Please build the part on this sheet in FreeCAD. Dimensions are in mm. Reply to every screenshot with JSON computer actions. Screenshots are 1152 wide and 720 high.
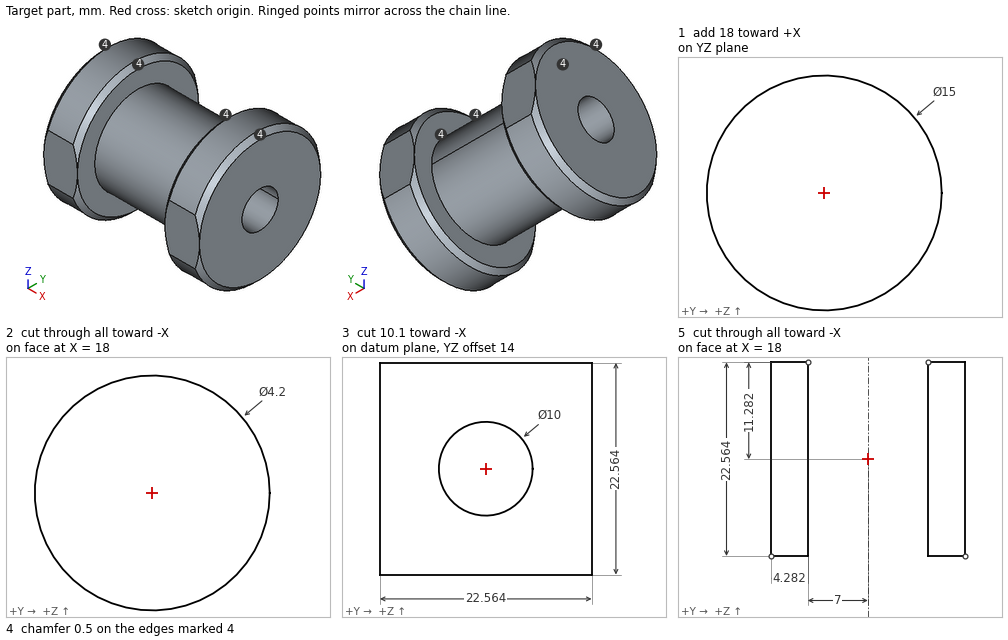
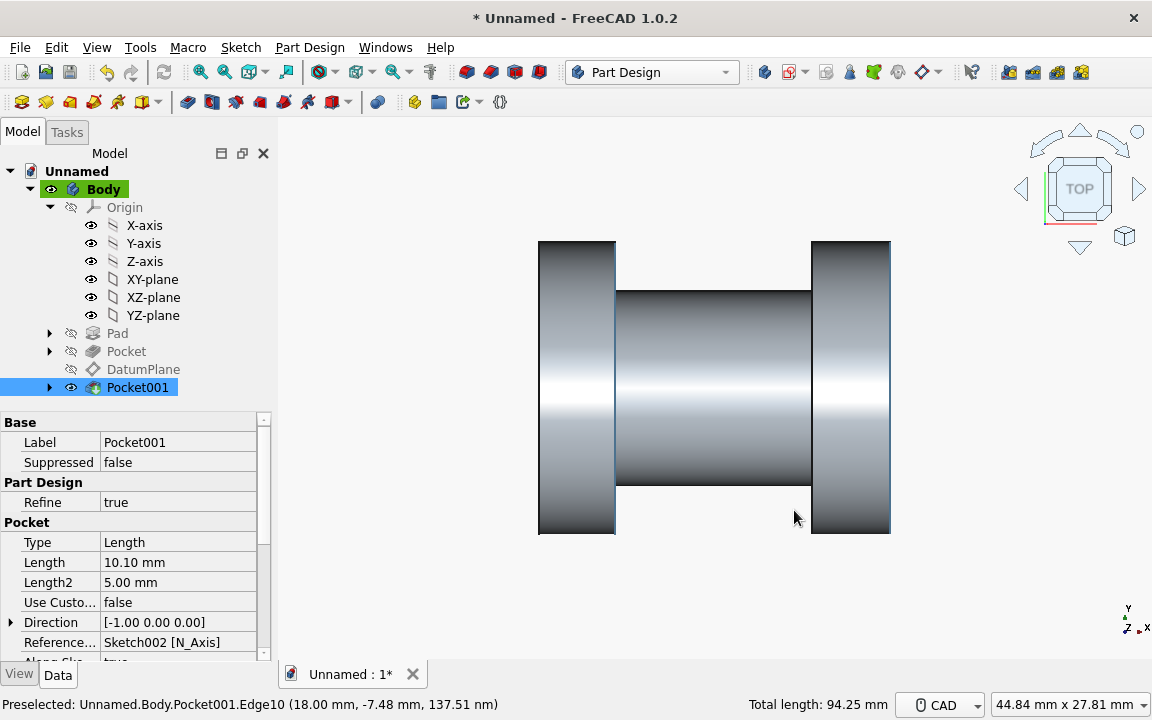
{"action": "left_click", "coordinate": [812, 505], "text": "ctrl"}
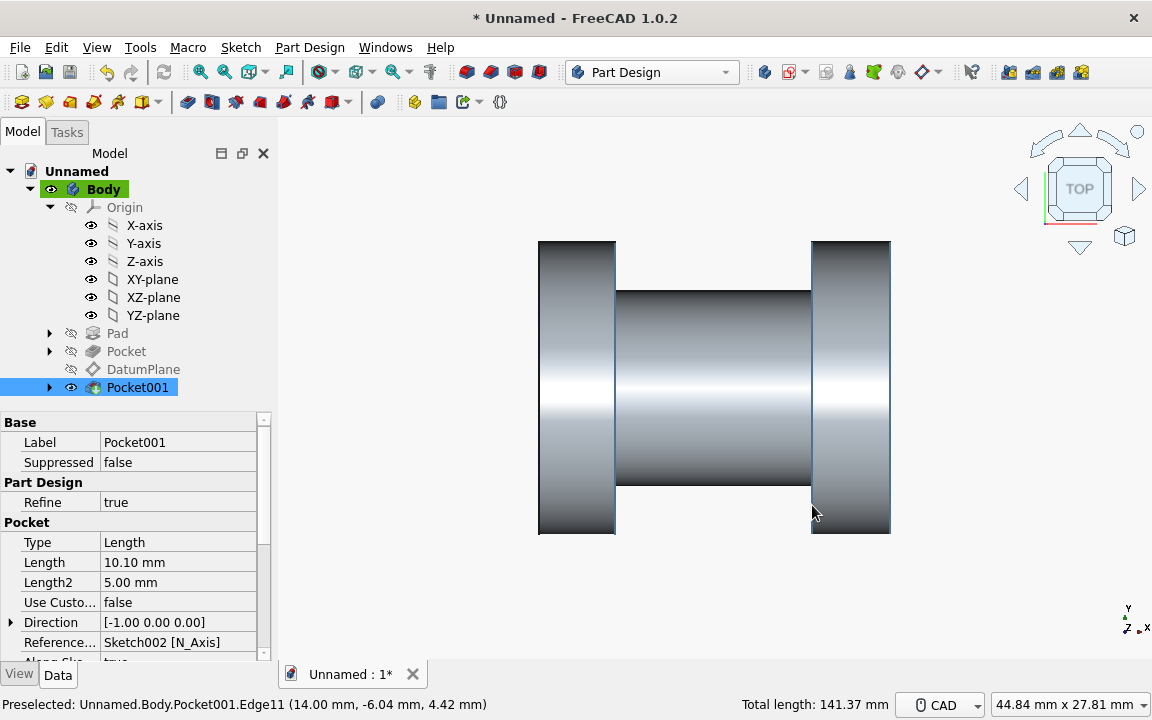
{"action": "left_click", "coordinate": [539, 505], "text": "ctrl"}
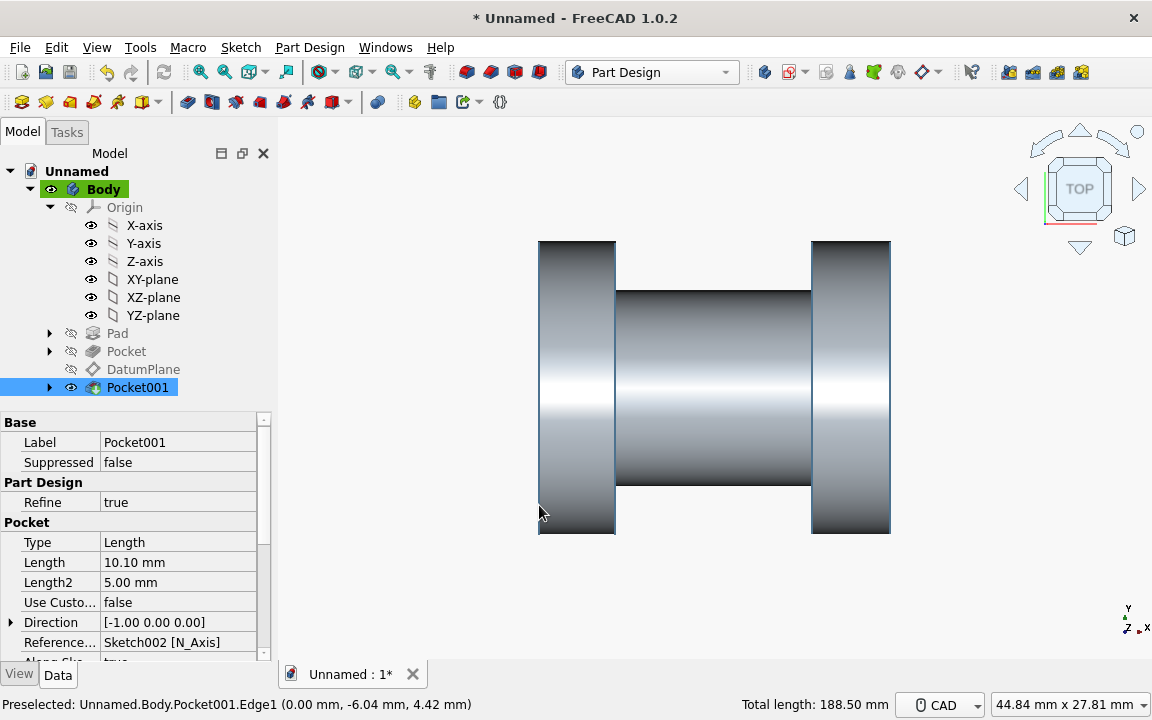
{"action": "left_click", "coordinate": [492, 72]}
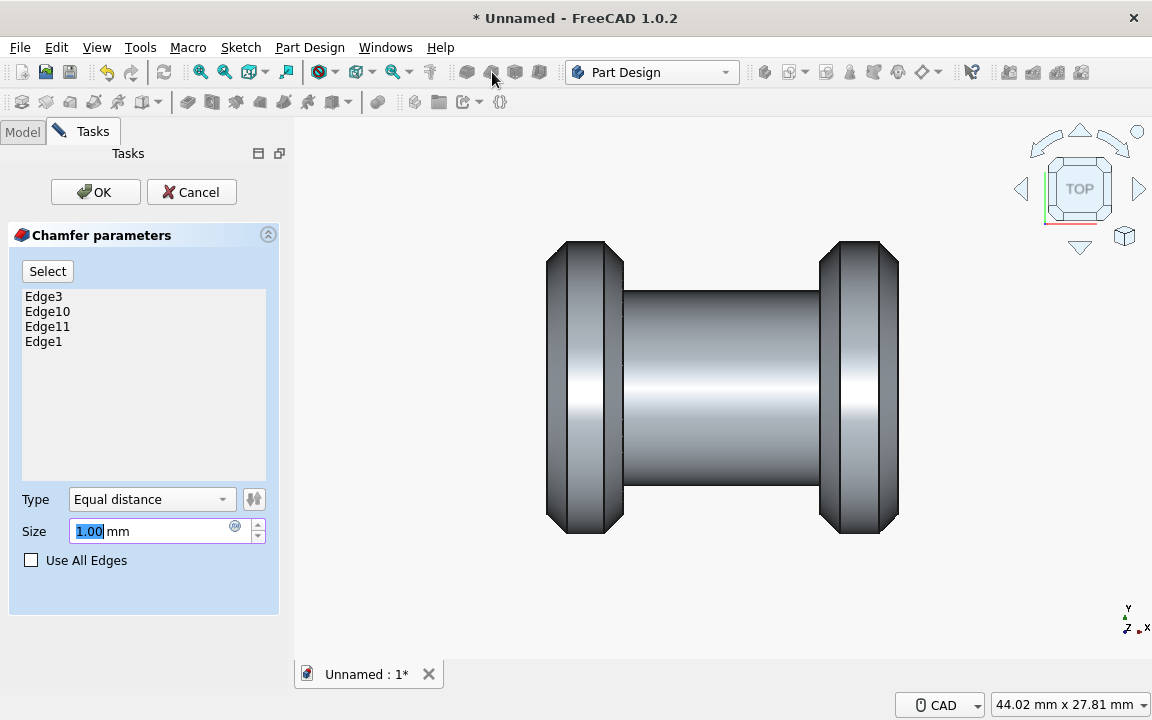
{"action": "type", "text": "0.5"}
{"action": "key", "text": "Tab"}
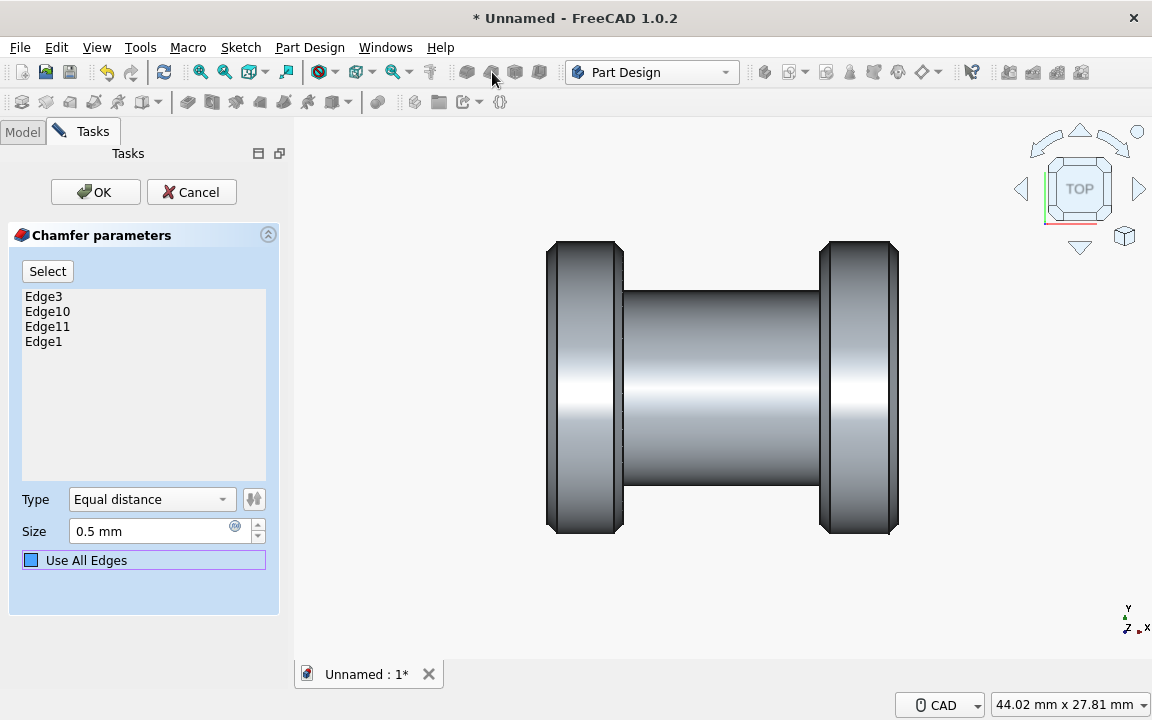
{"action": "left_click", "coordinate": [96, 192]}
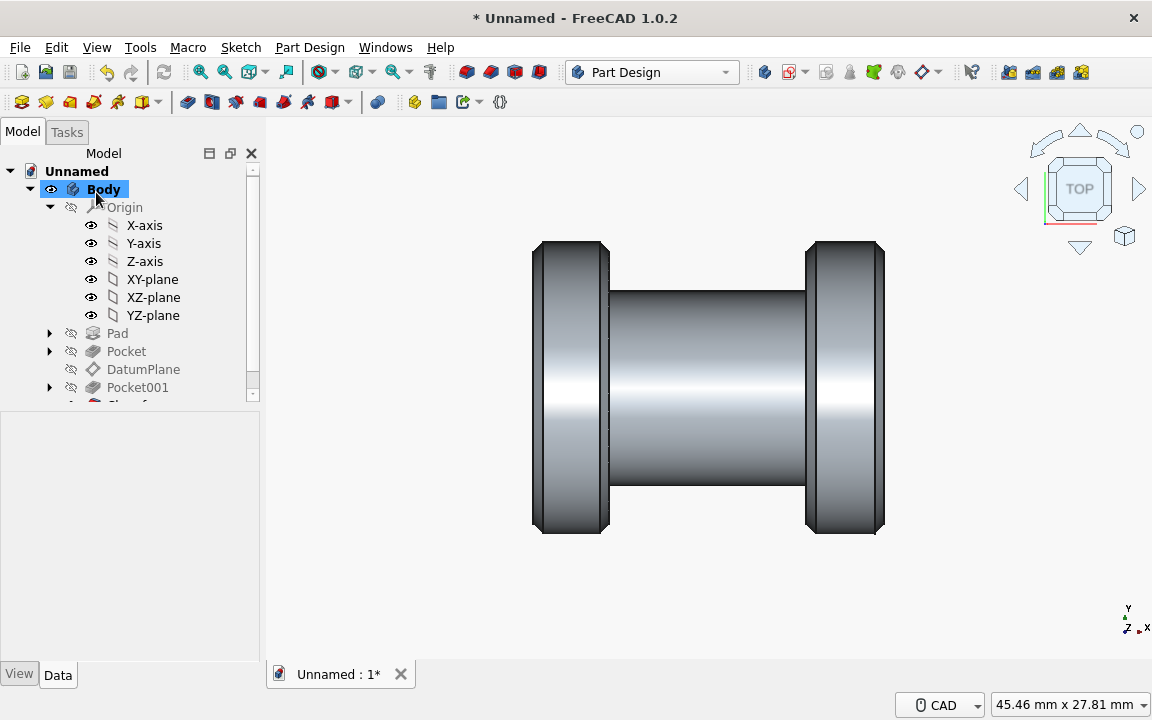
{"action": "key", "text": "0"}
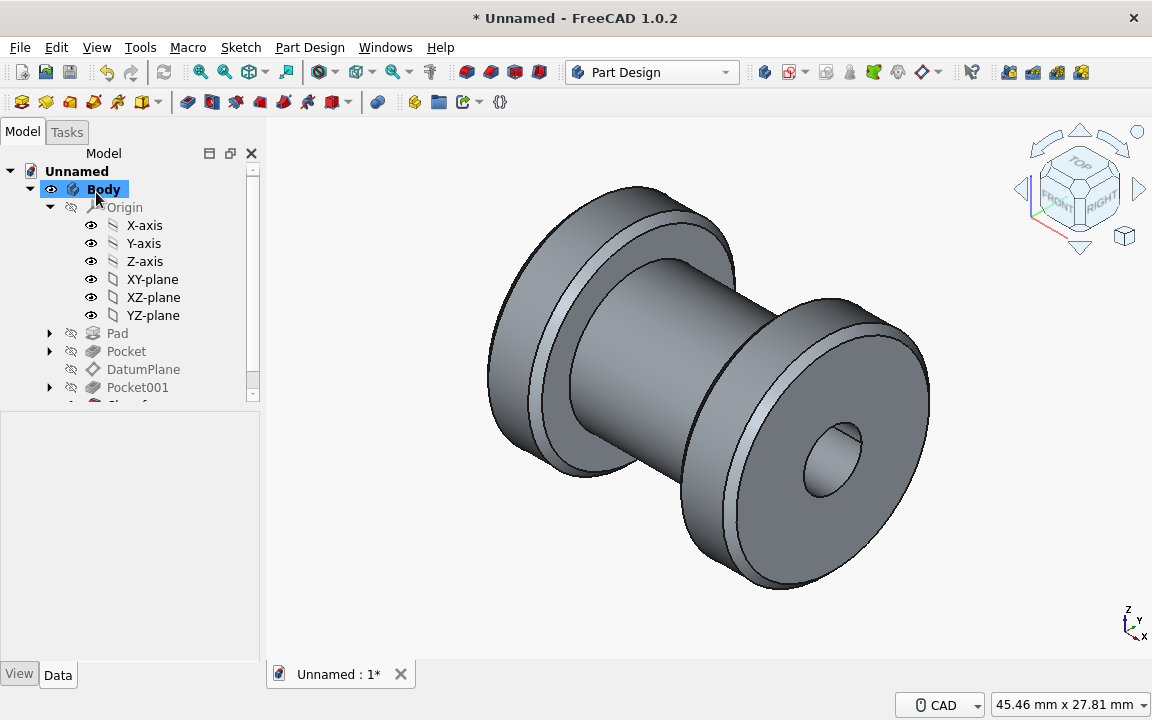
{"action": "left_click", "coordinate": [888, 395]}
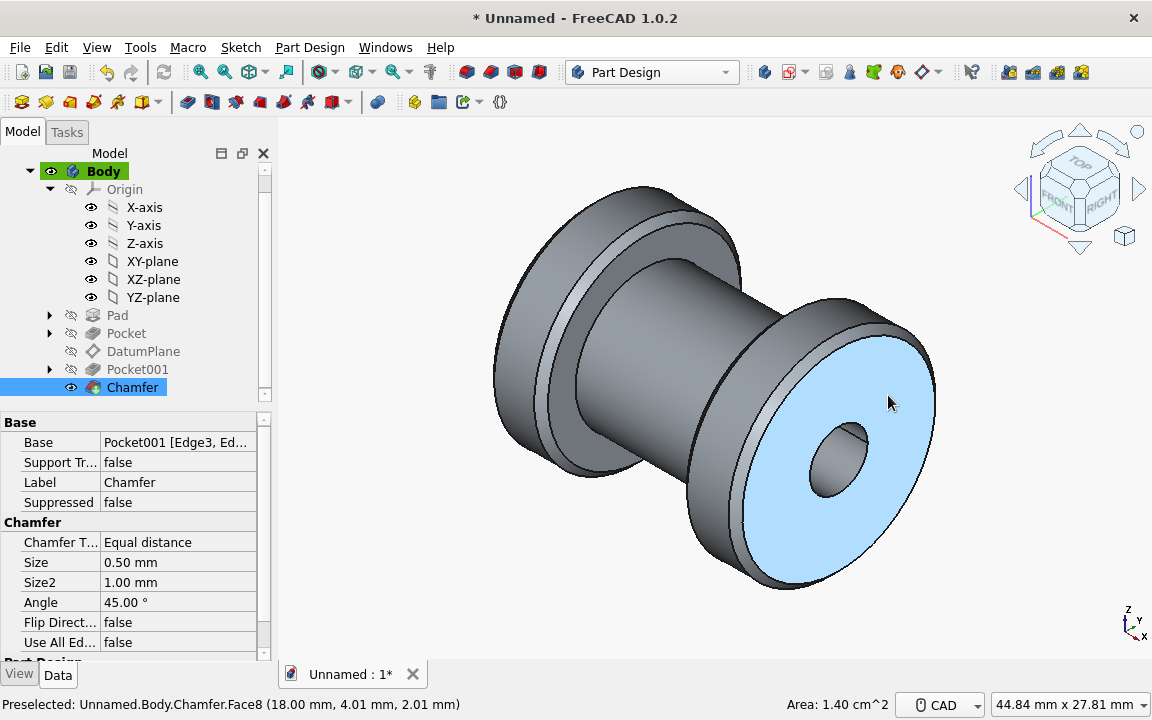
{"action": "left_click", "coordinate": [790, 72]}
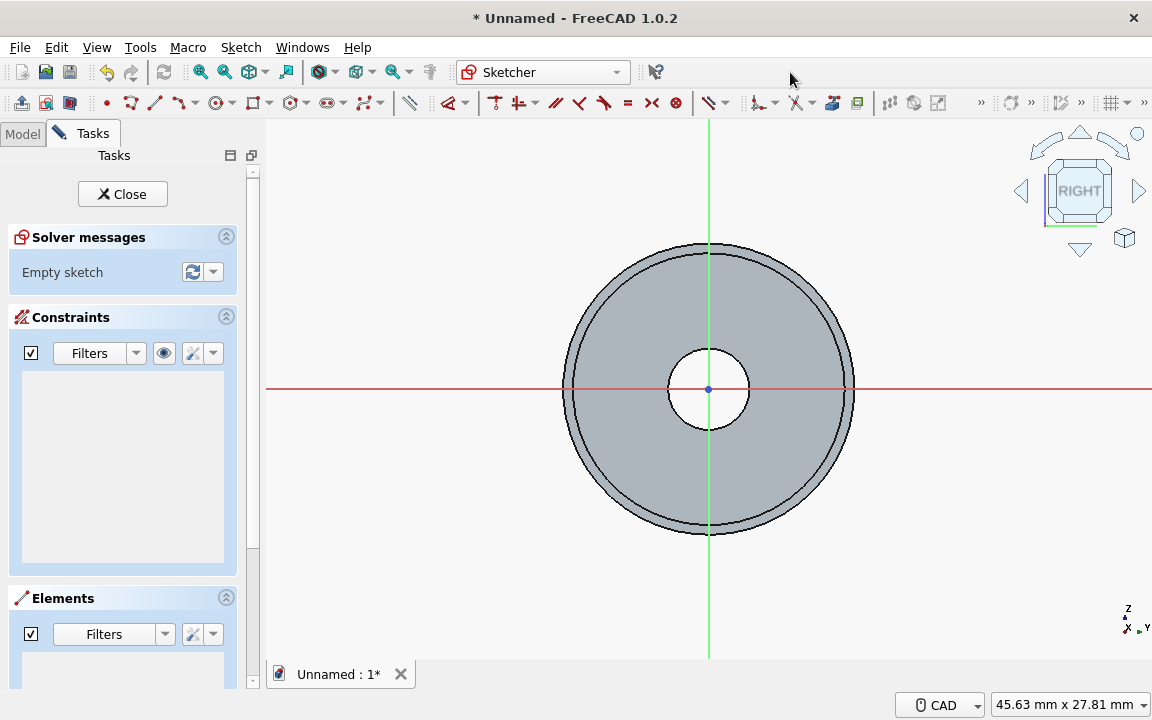
{"action": "scroll", "coordinate": [332, 388], "scroll_direction": "down", "scroll_amount": 1}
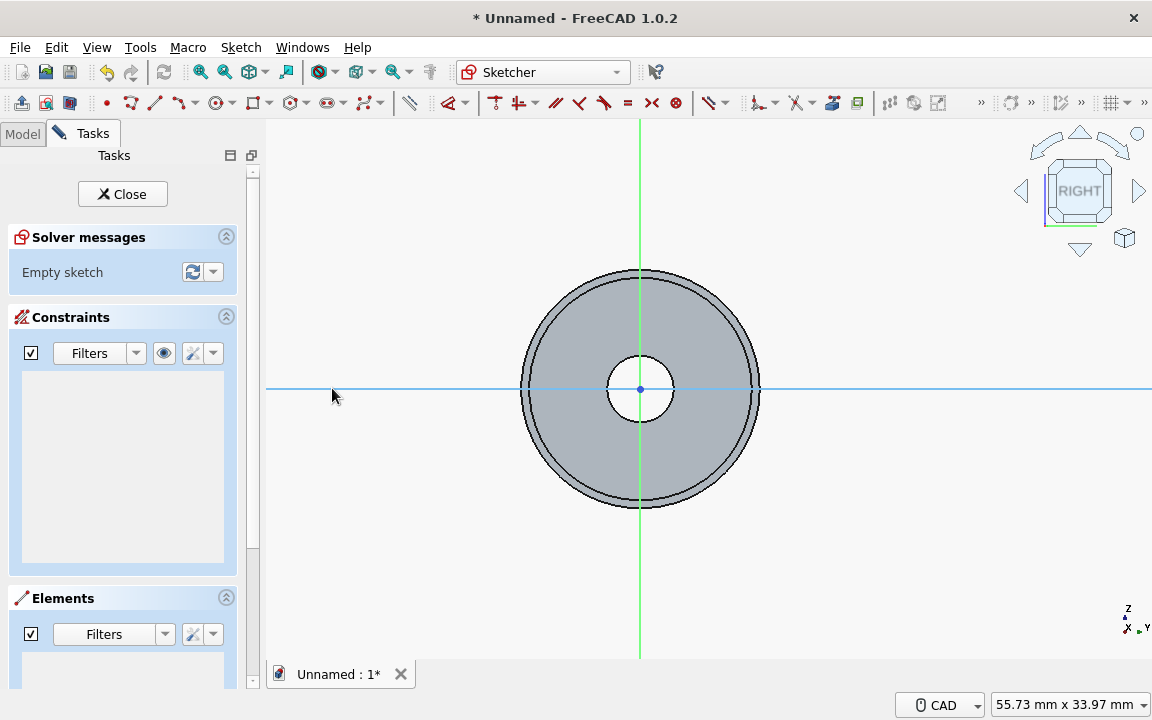
{"action": "left_click", "coordinate": [254, 104]}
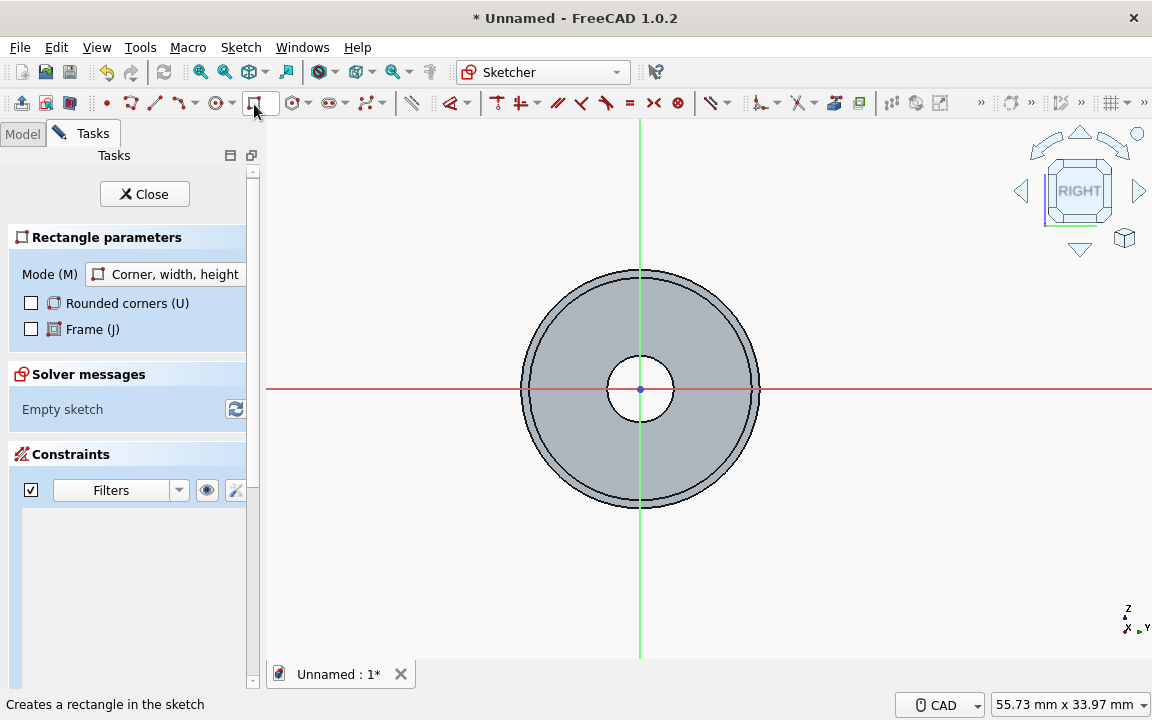
{"action": "left_click", "coordinate": [461, 210]}
{"action": "left_click", "coordinate": [529, 568]}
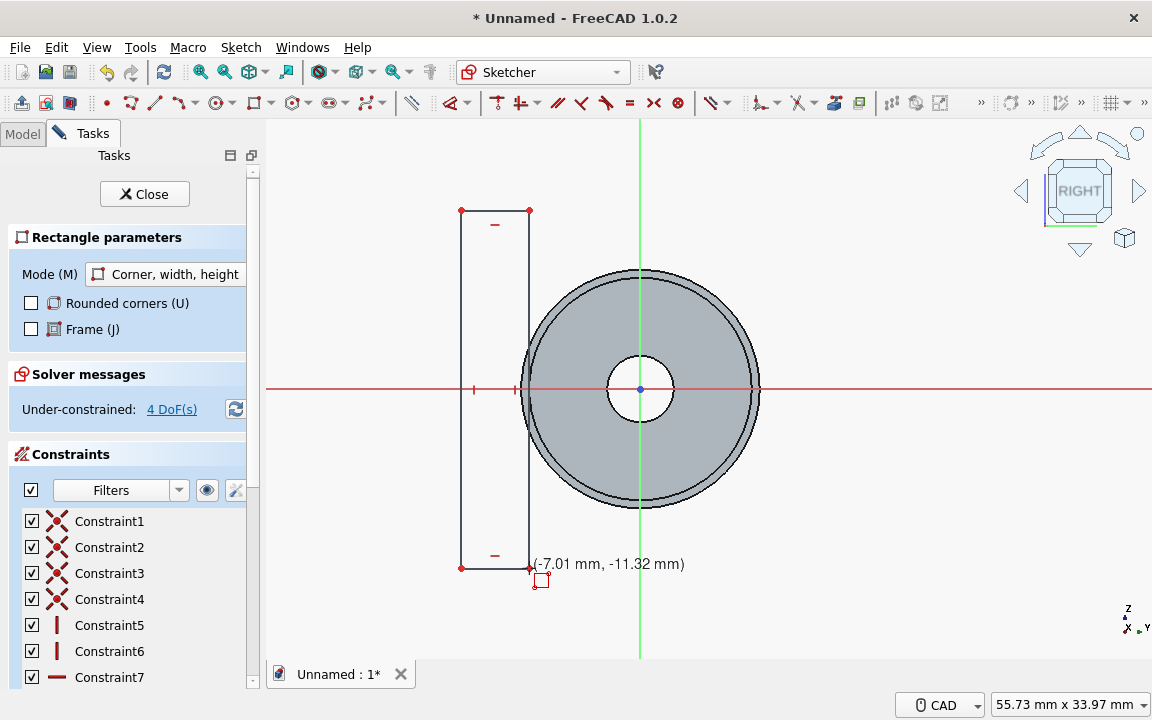
{"action": "left_click", "coordinate": [752, 210]}
{"action": "left_click", "coordinate": [820, 568]}
{"action": "key", "text": "Escape"}